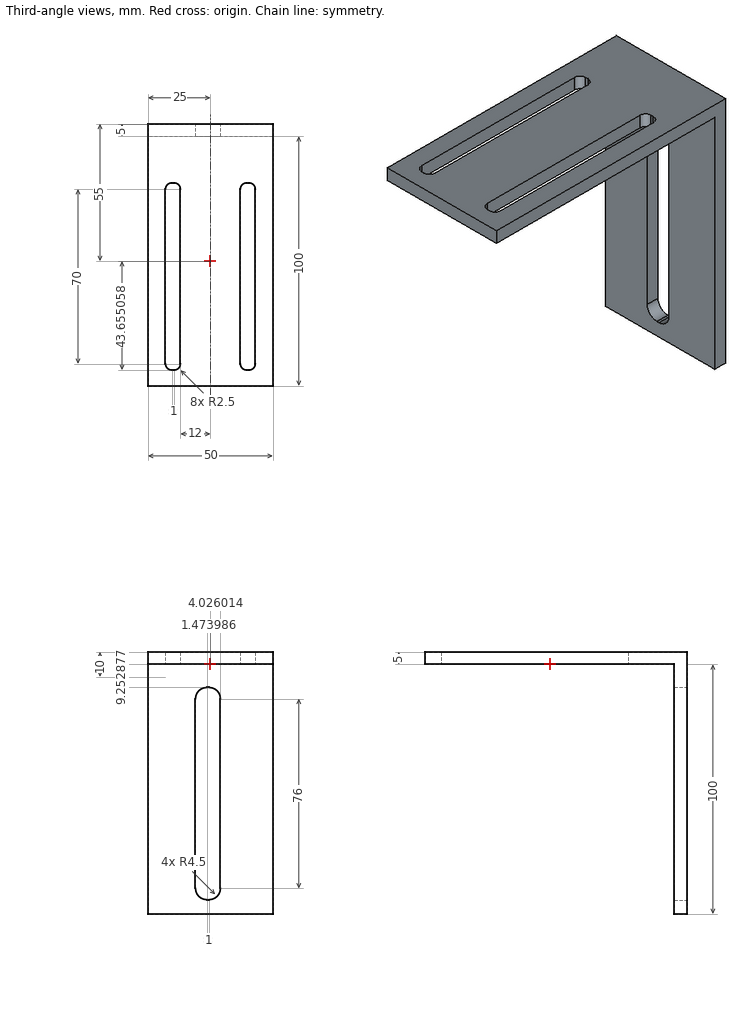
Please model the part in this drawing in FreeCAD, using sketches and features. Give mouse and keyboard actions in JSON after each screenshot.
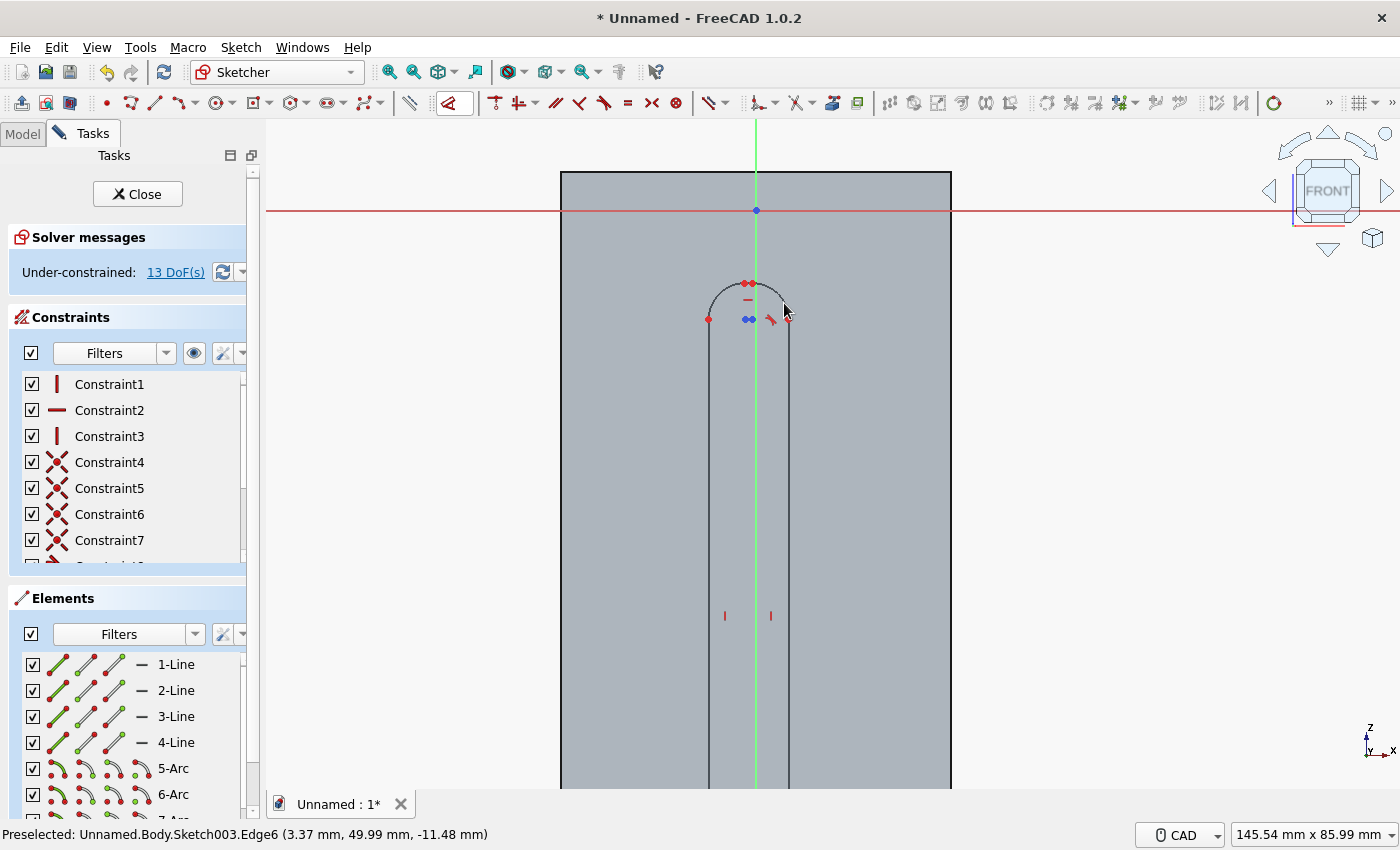
{"action": "scroll", "coordinate": [749, 283], "scroll_direction": "up", "scroll_amount": 7}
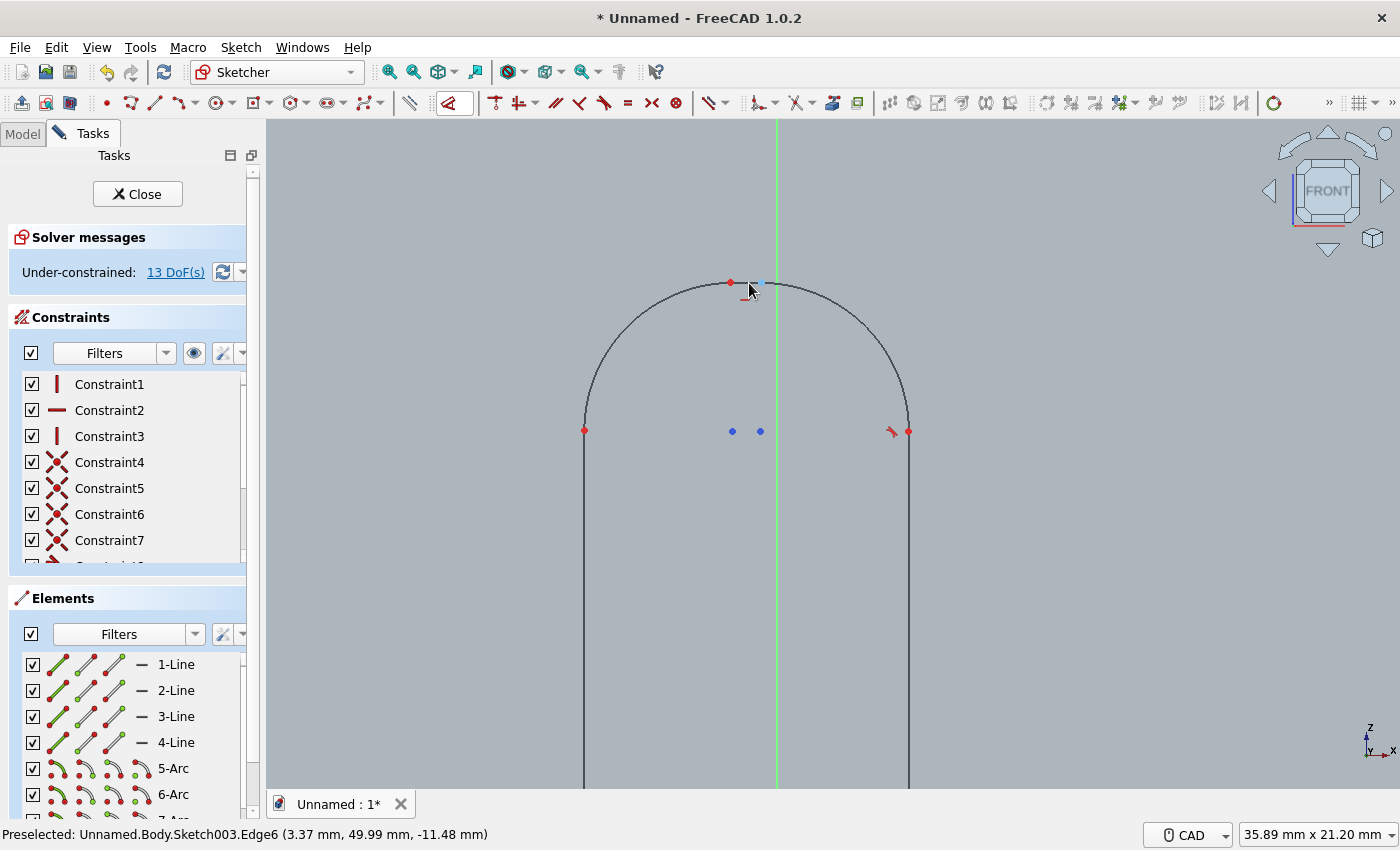
{"action": "left_click", "coordinate": [746, 283]}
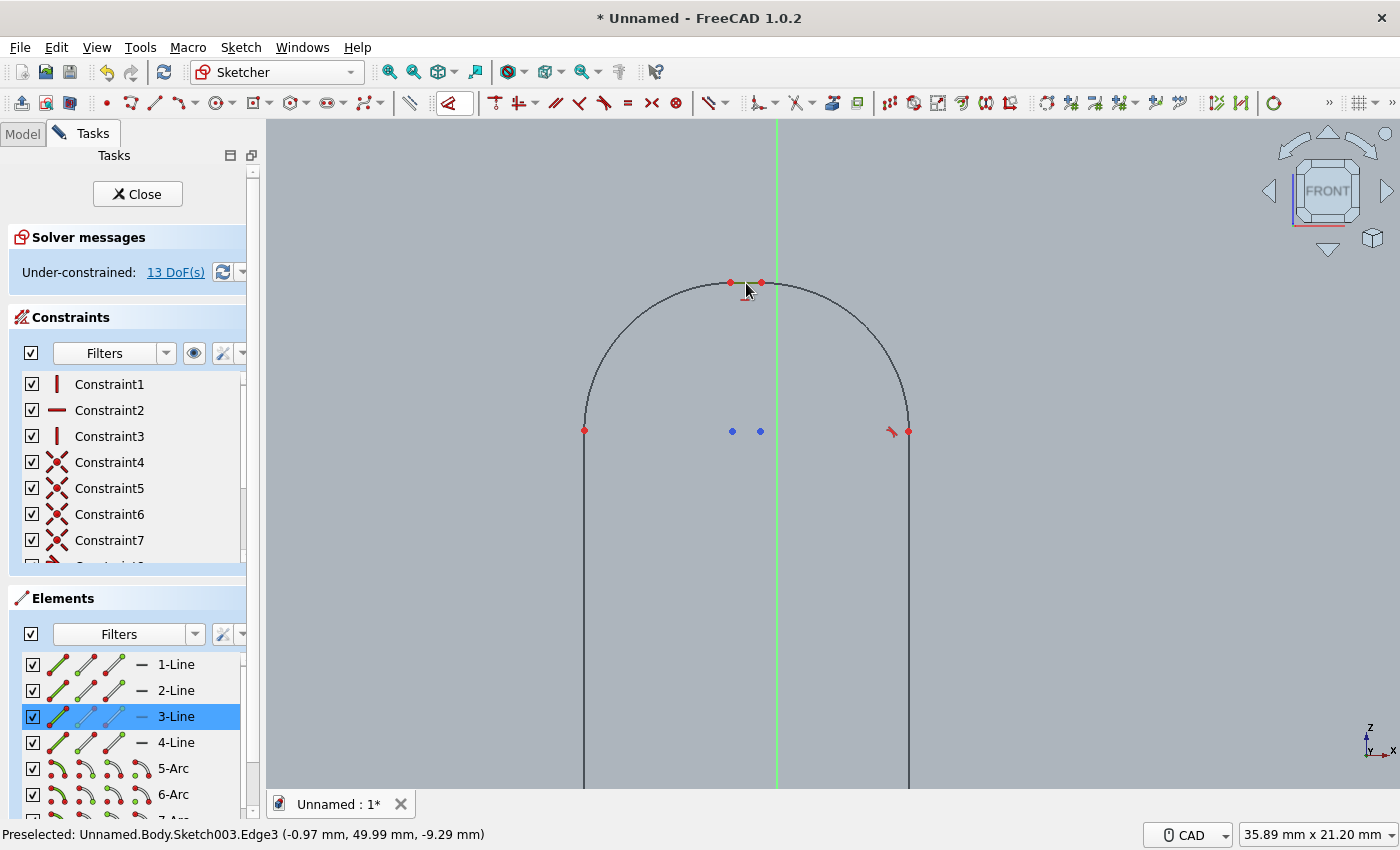
{"action": "scroll", "coordinate": [767, 294], "scroll_direction": "down", "scroll_amount": 10}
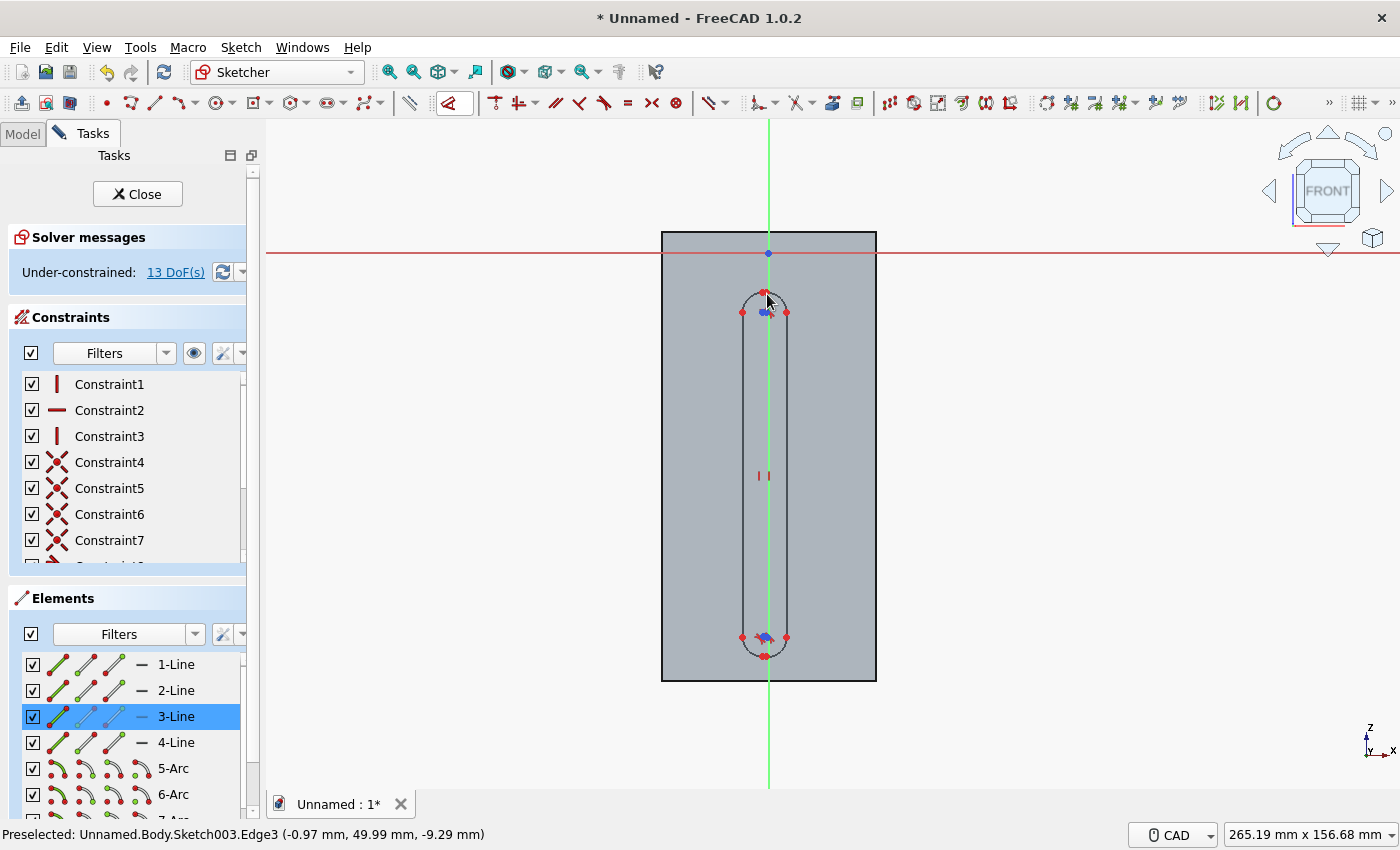
{"action": "scroll", "coordinate": [784, 304], "scroll_direction": "up", "scroll_amount": 2}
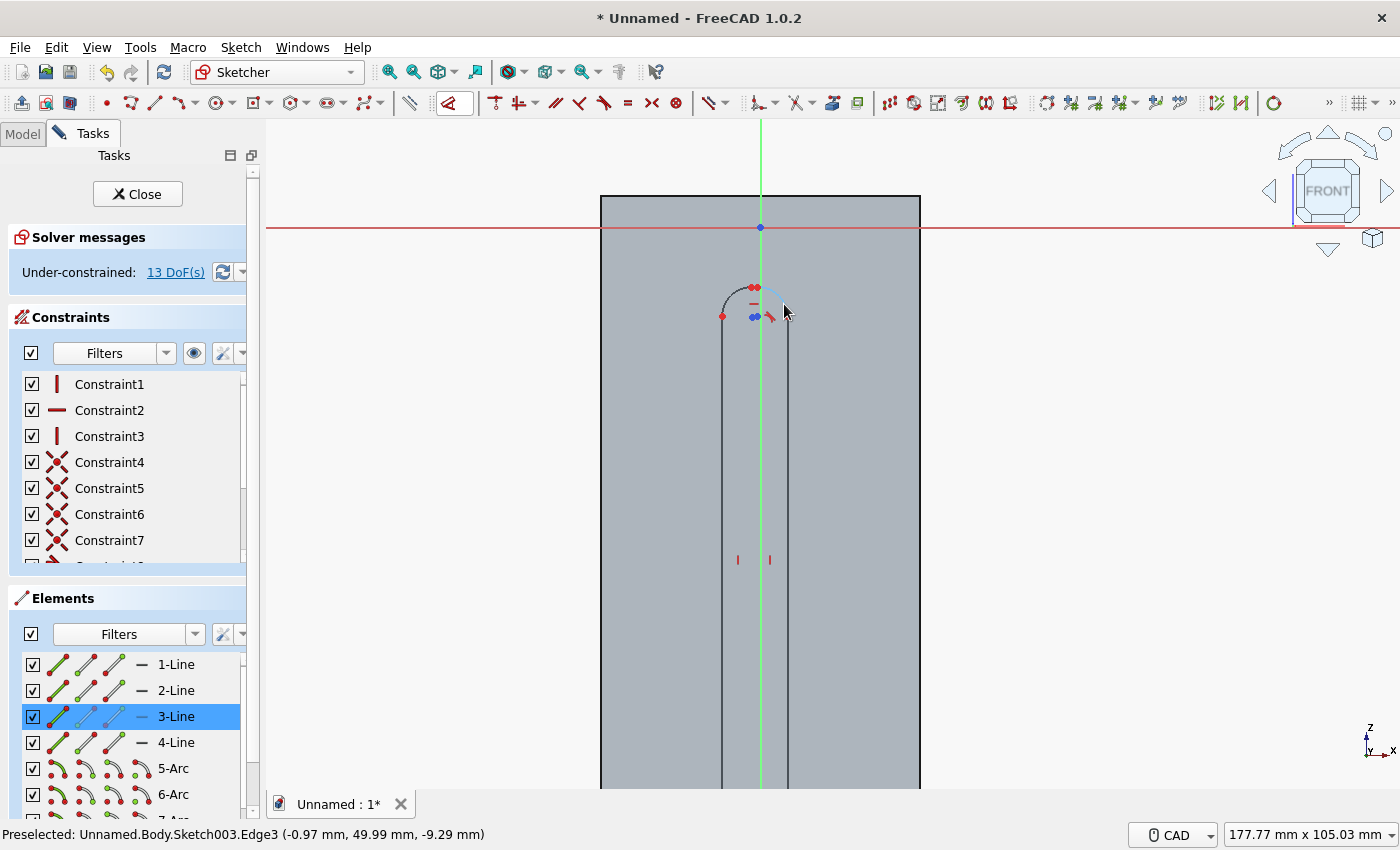
{"action": "left_click", "coordinate": [784, 303]}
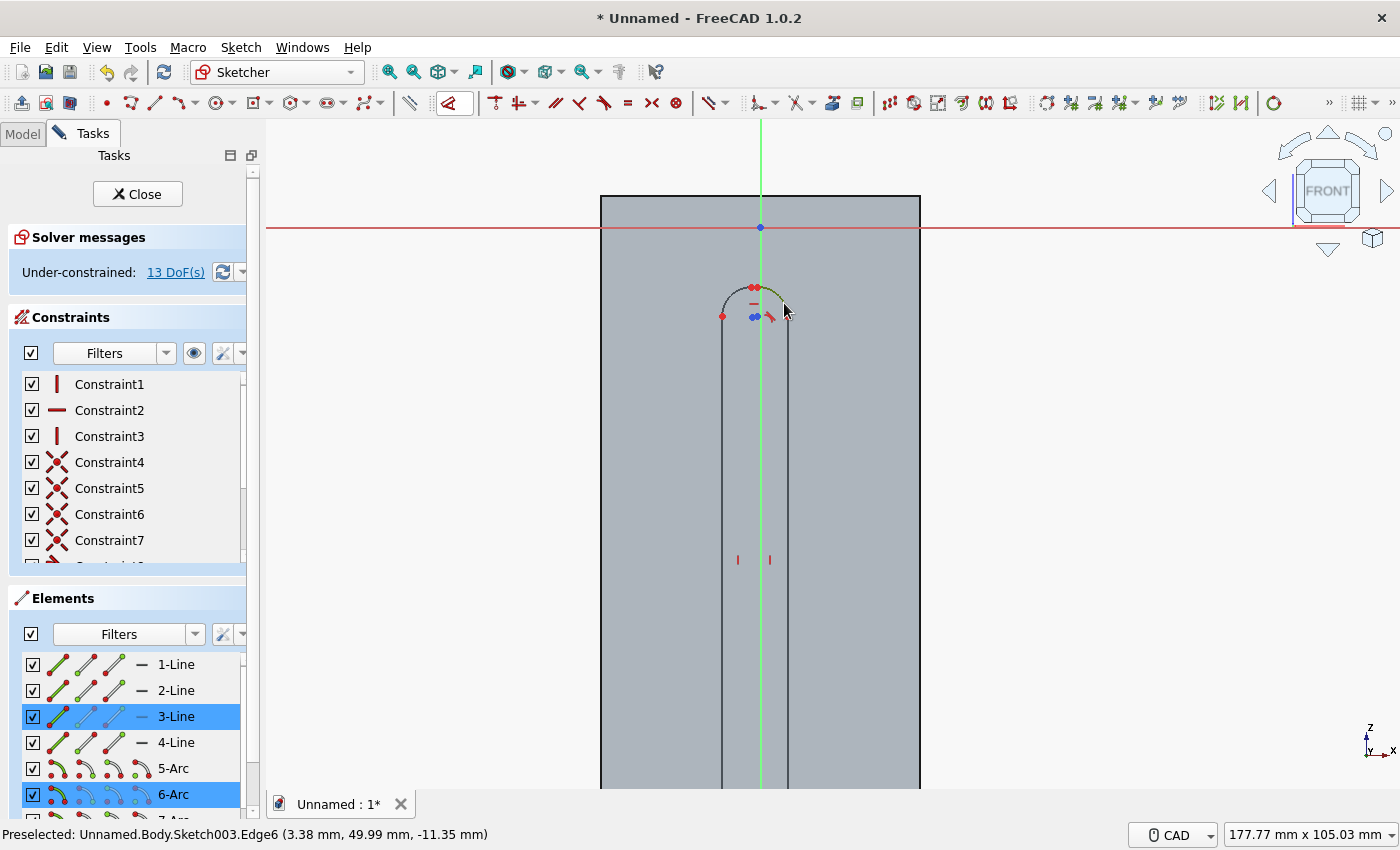
{"action": "left_click", "coordinate": [604, 104]}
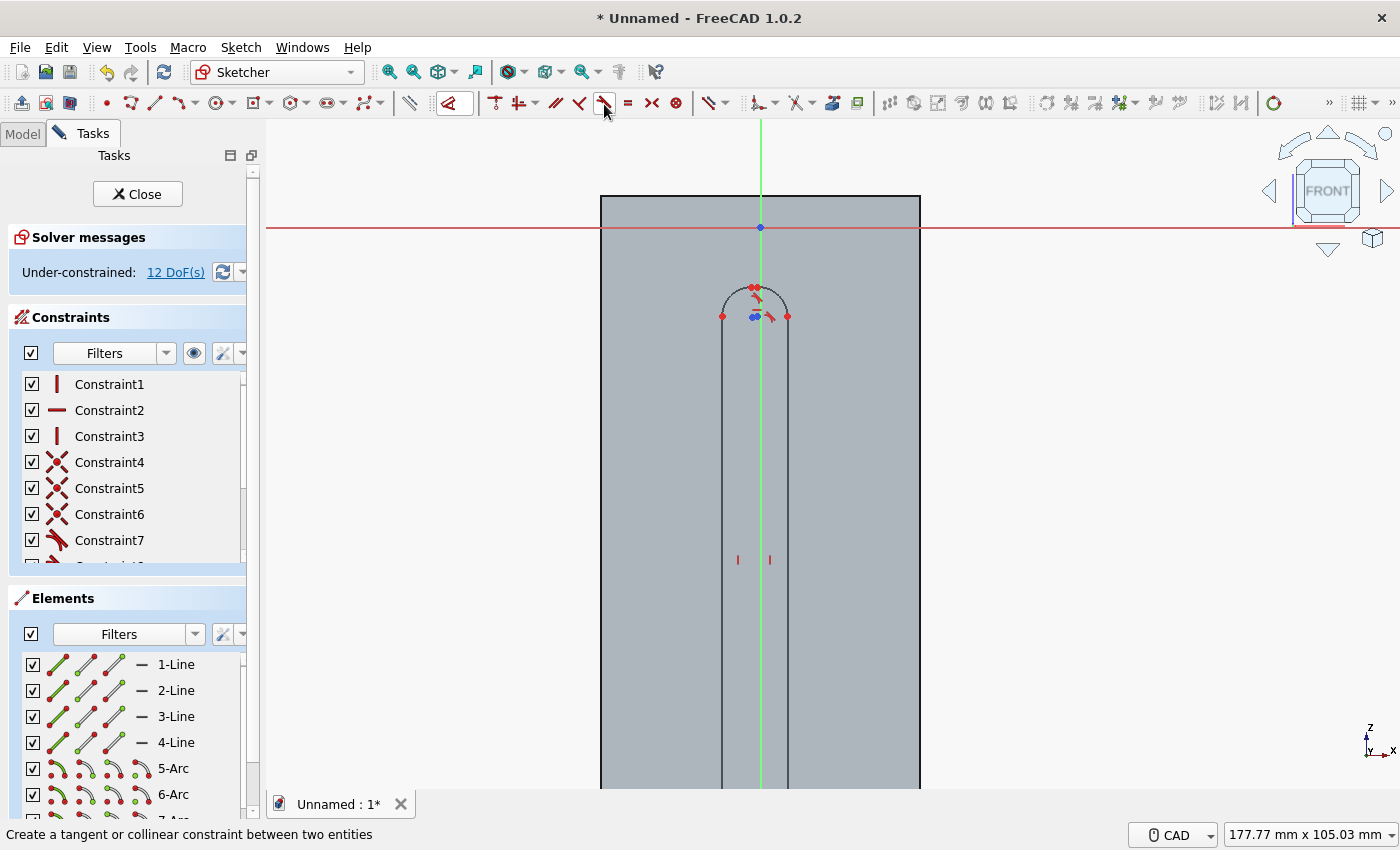
{"action": "scroll", "coordinate": [755, 287], "scroll_direction": "up", "scroll_amount": 8}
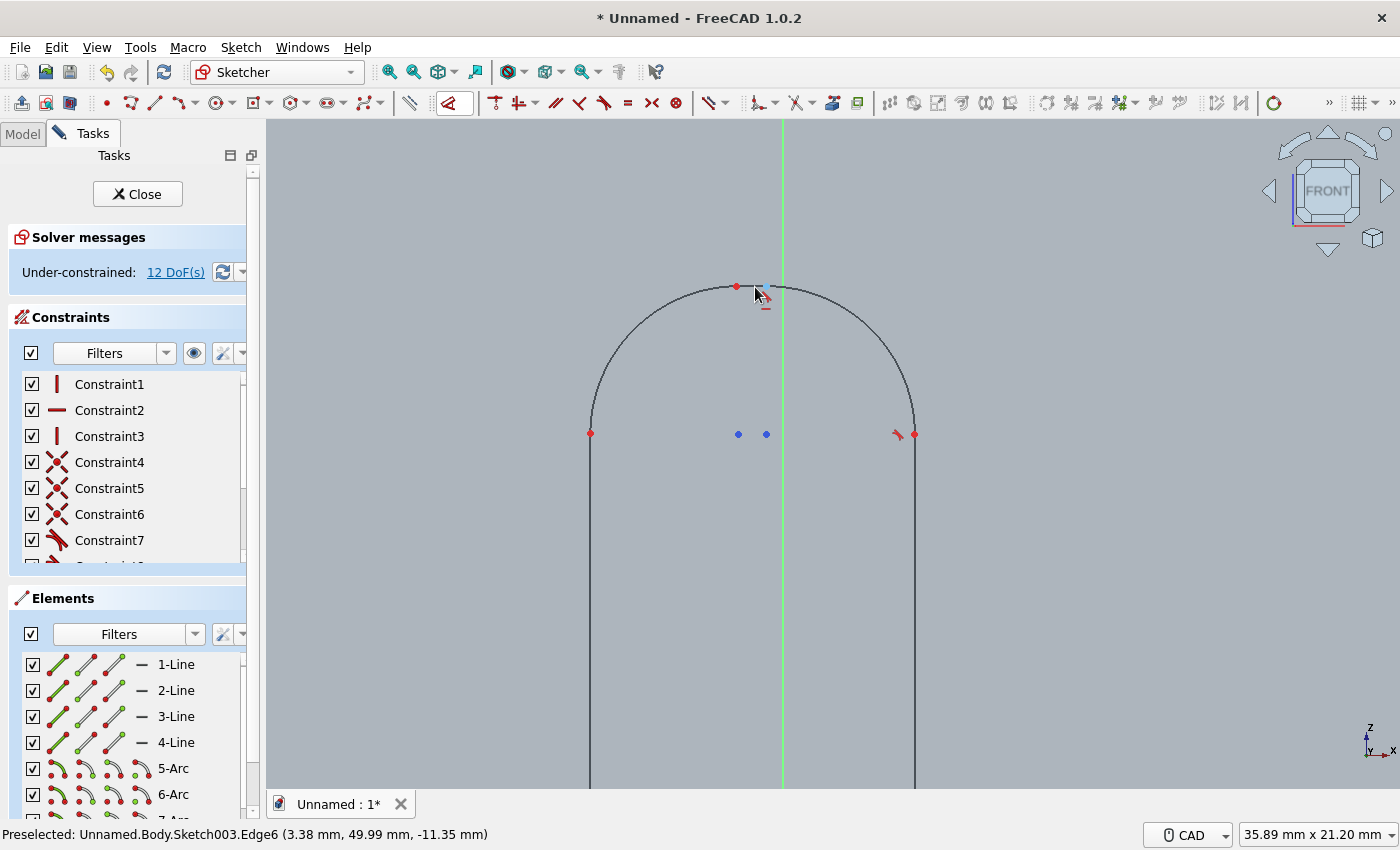
{"action": "left_click", "coordinate": [751, 286]}